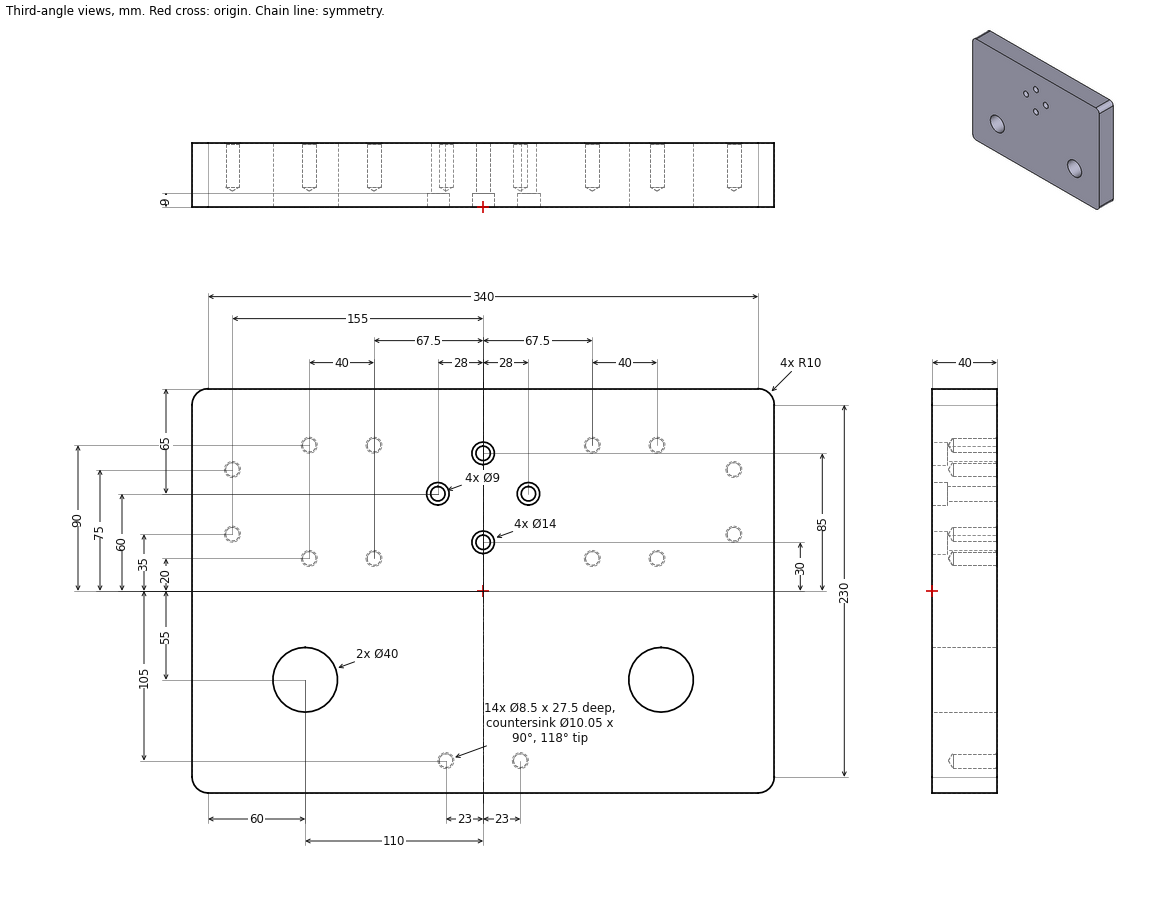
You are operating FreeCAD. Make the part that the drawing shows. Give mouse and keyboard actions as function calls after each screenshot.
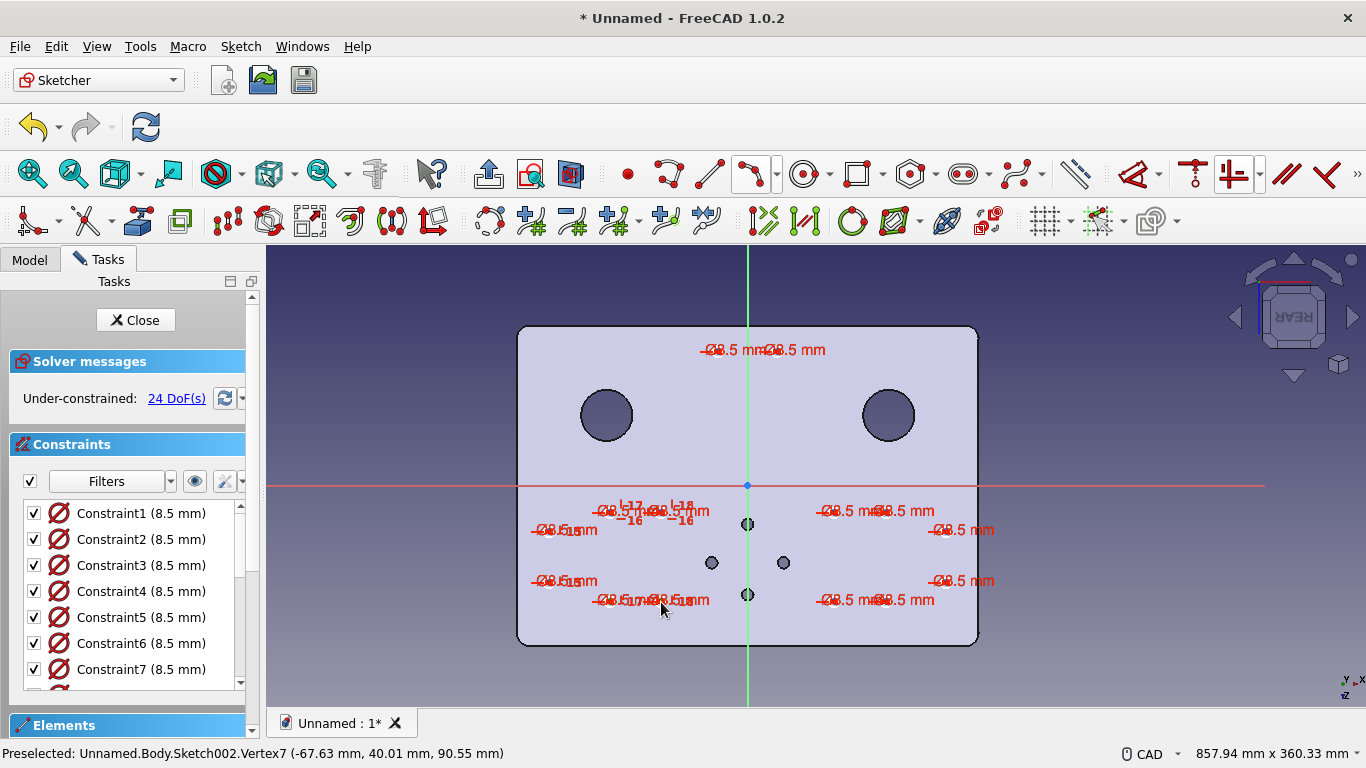
key(h)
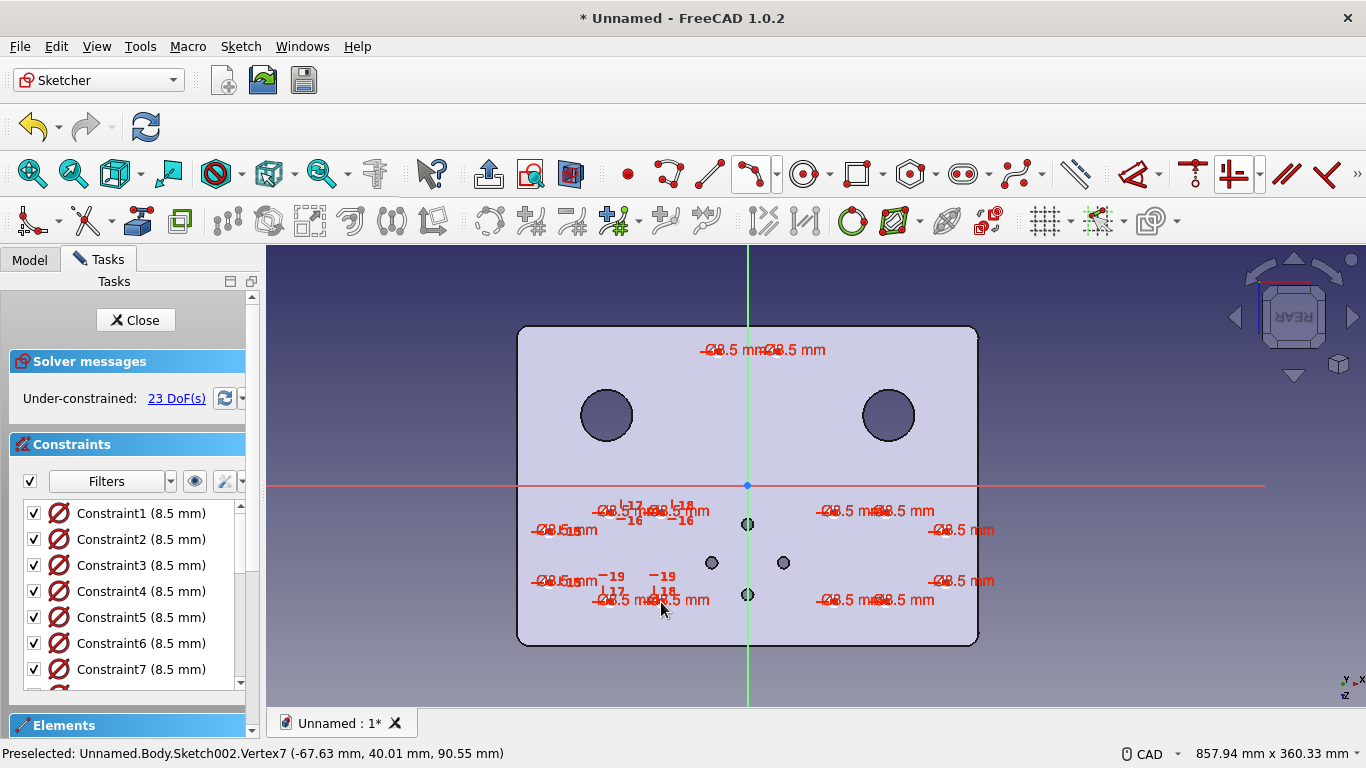
click(549, 583)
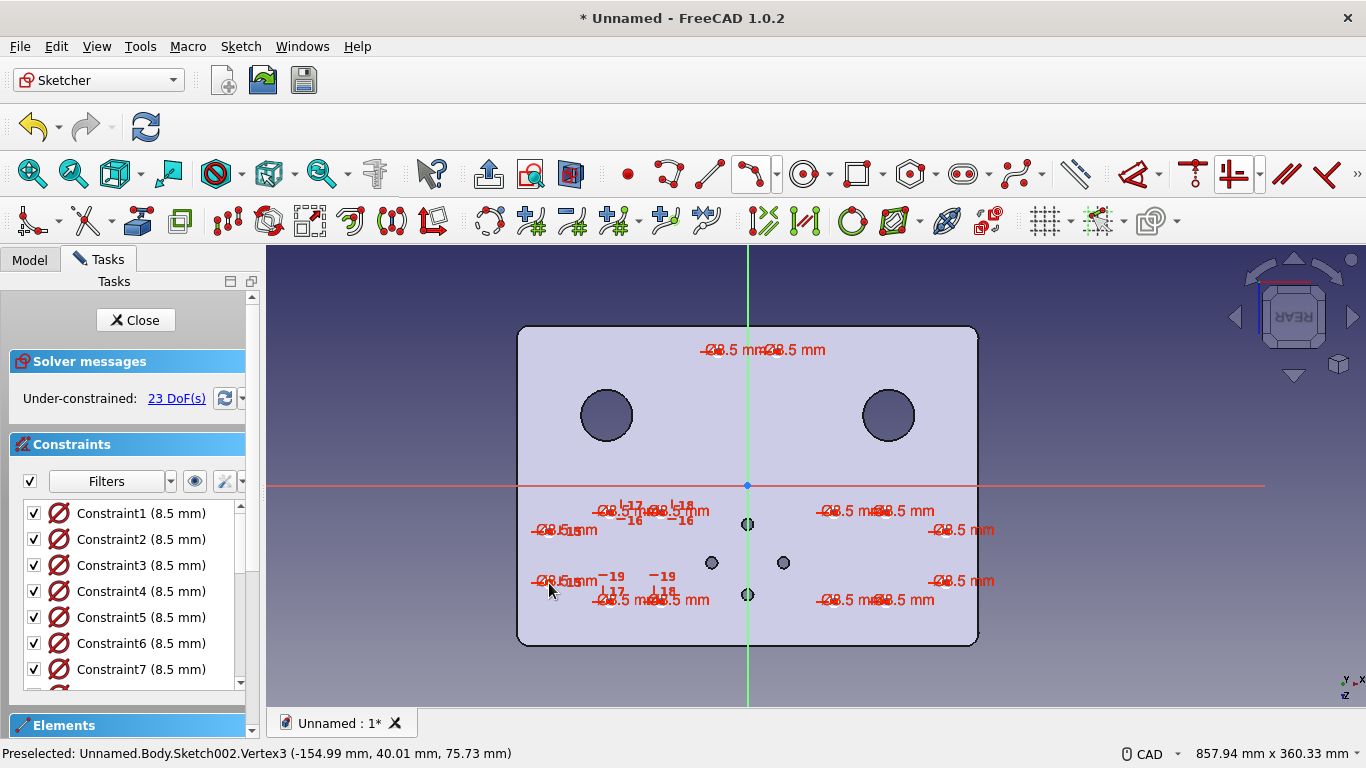
click(946, 583)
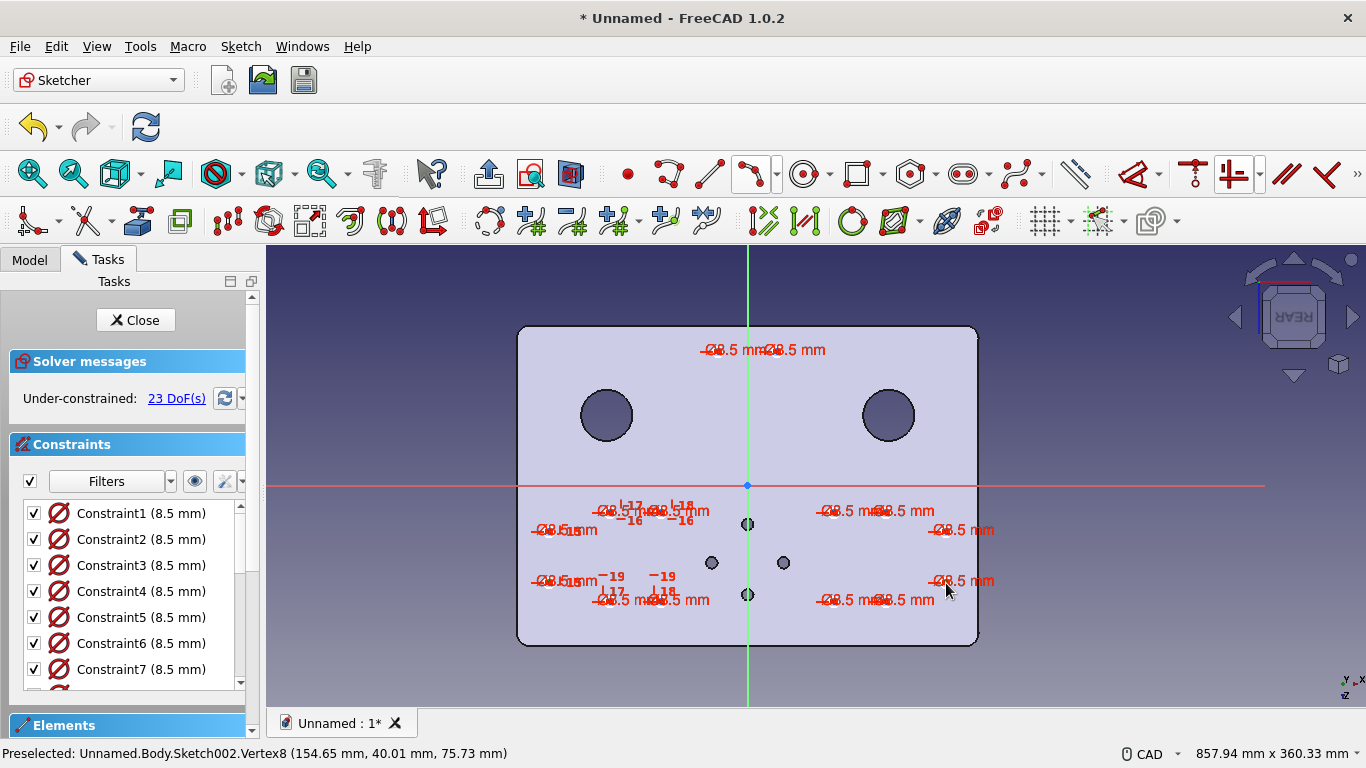
click(1260, 174)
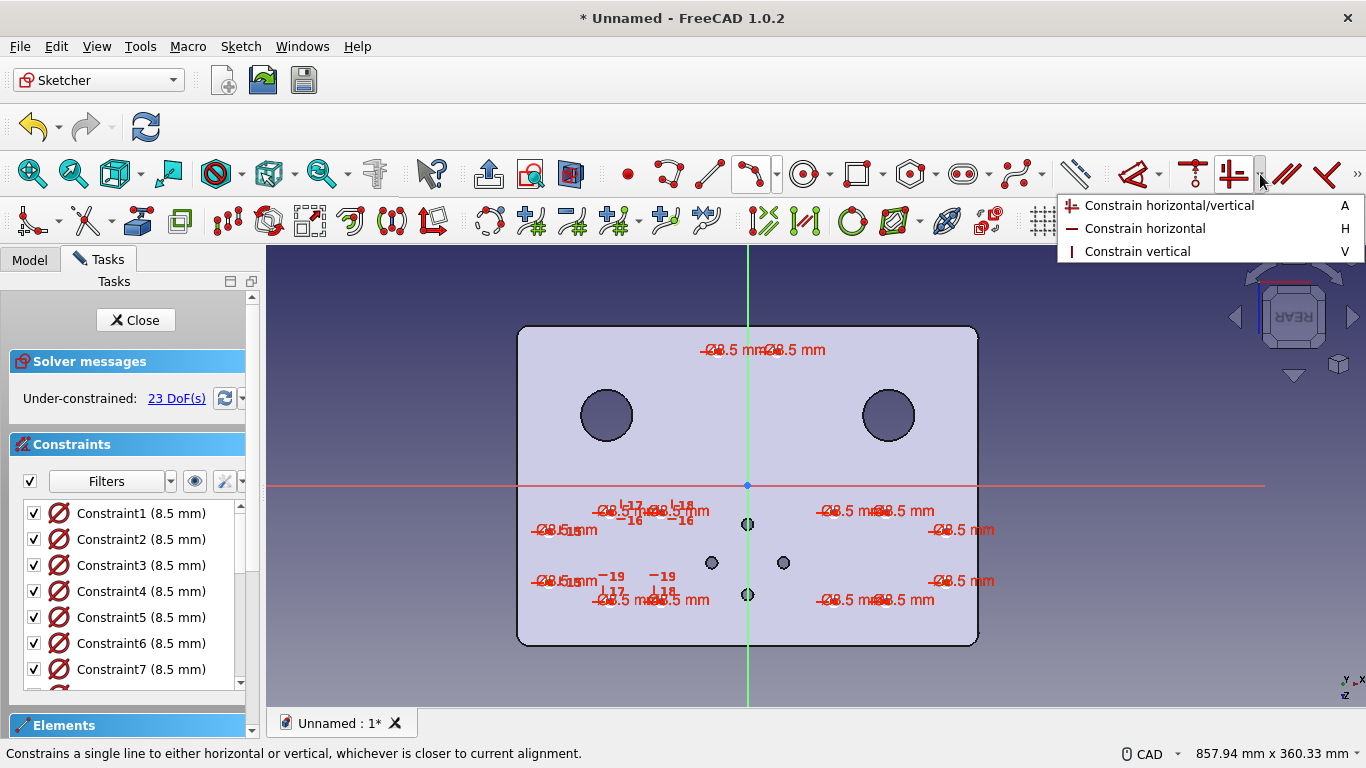
click(1211, 228)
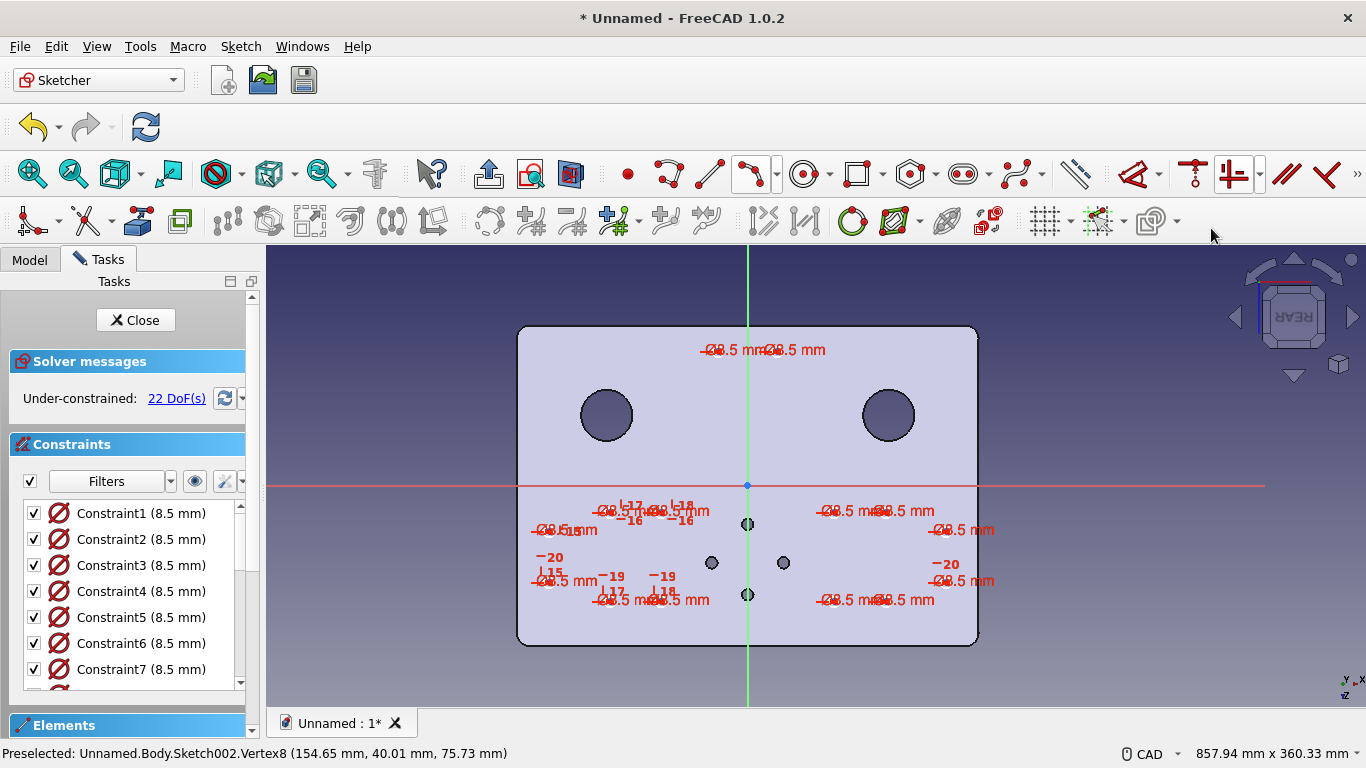
click(946, 583)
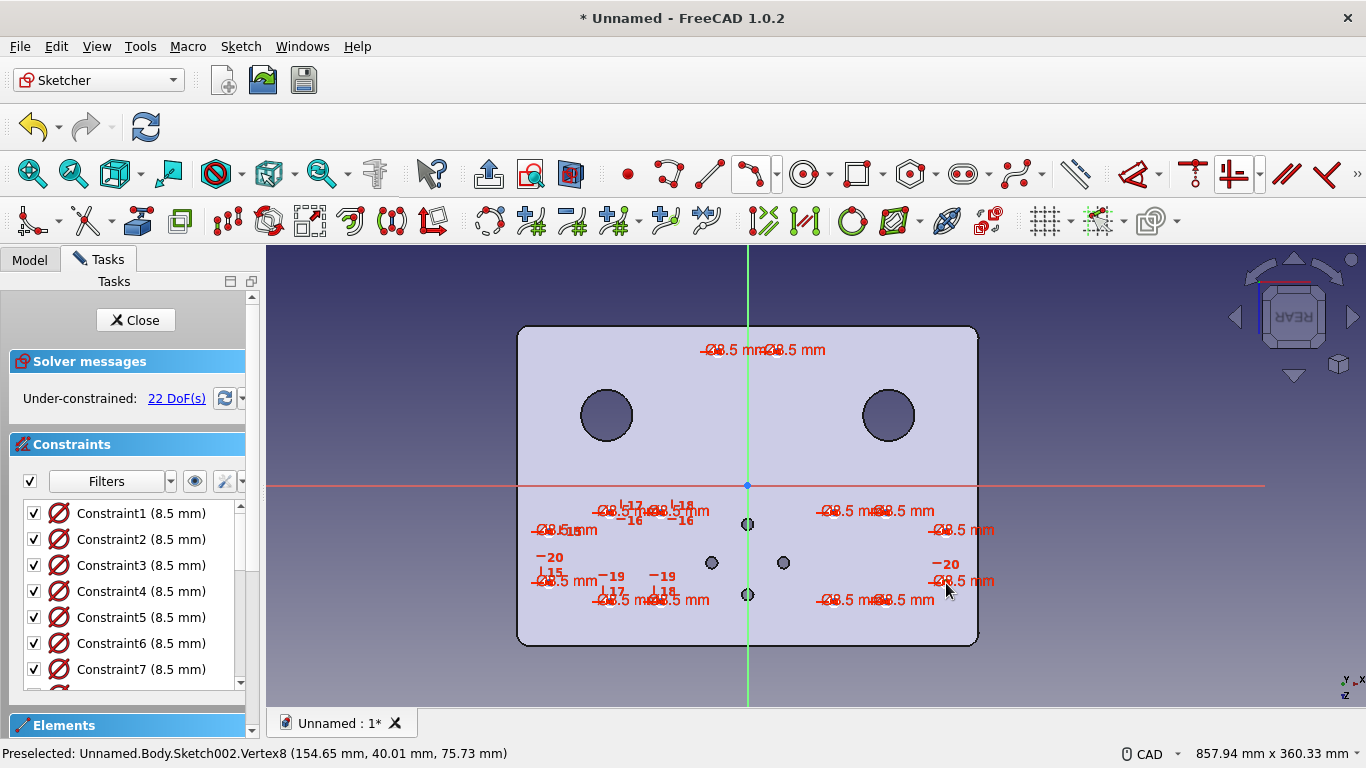
click(946, 532)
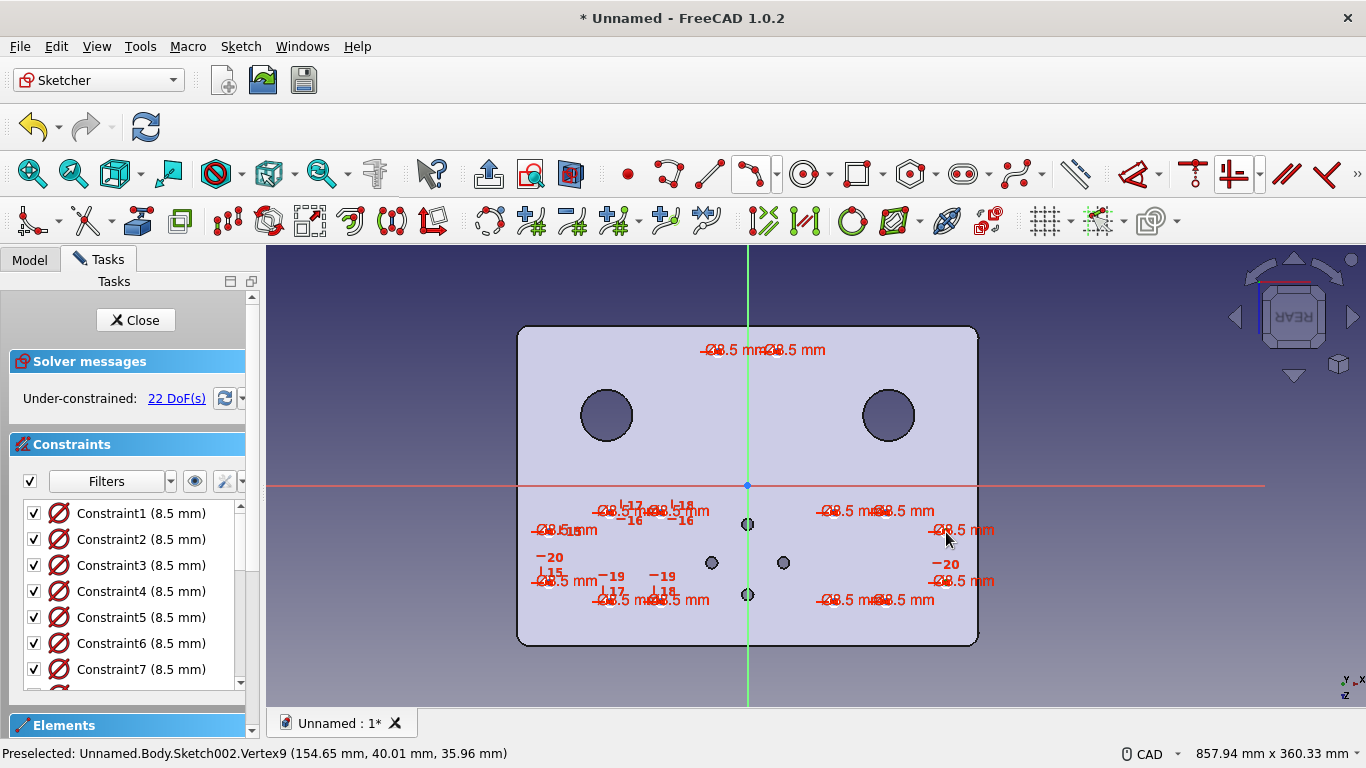
click(1260, 174)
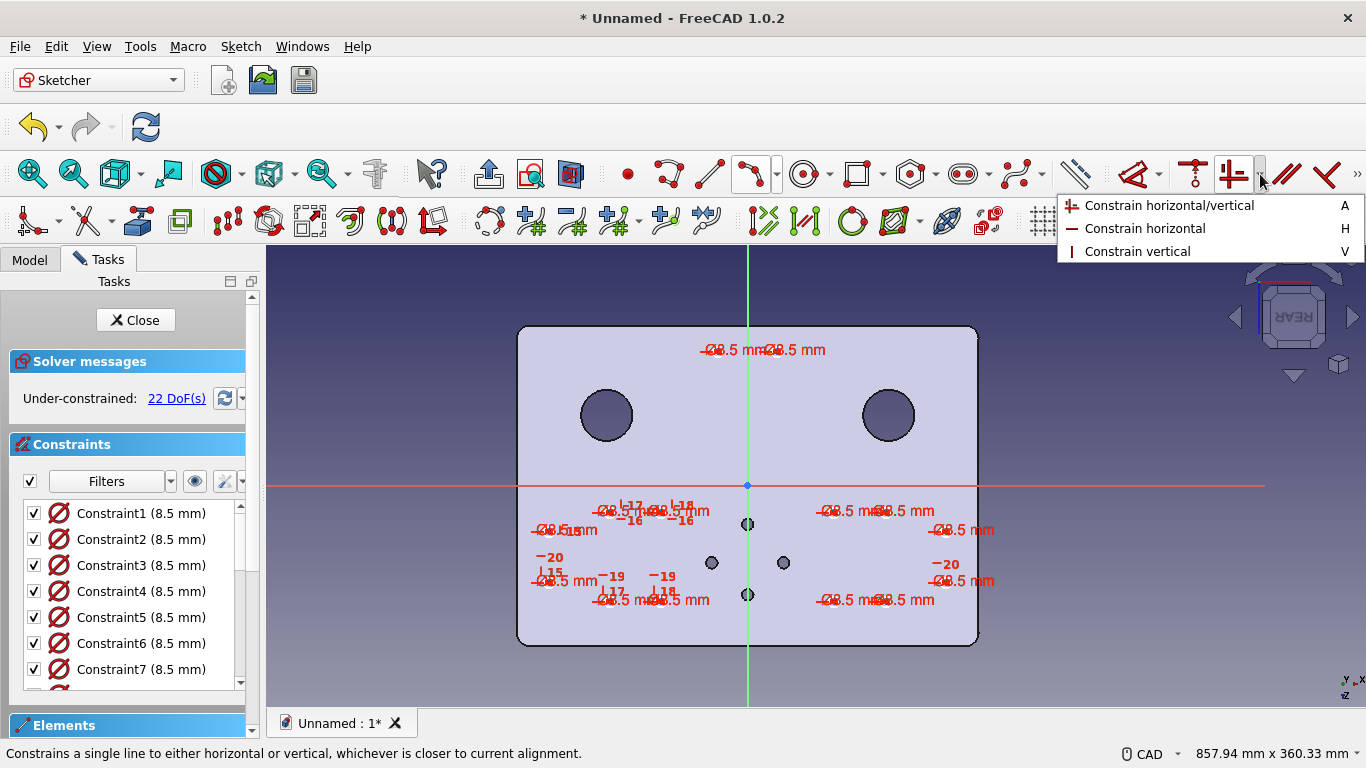
click(1211, 252)